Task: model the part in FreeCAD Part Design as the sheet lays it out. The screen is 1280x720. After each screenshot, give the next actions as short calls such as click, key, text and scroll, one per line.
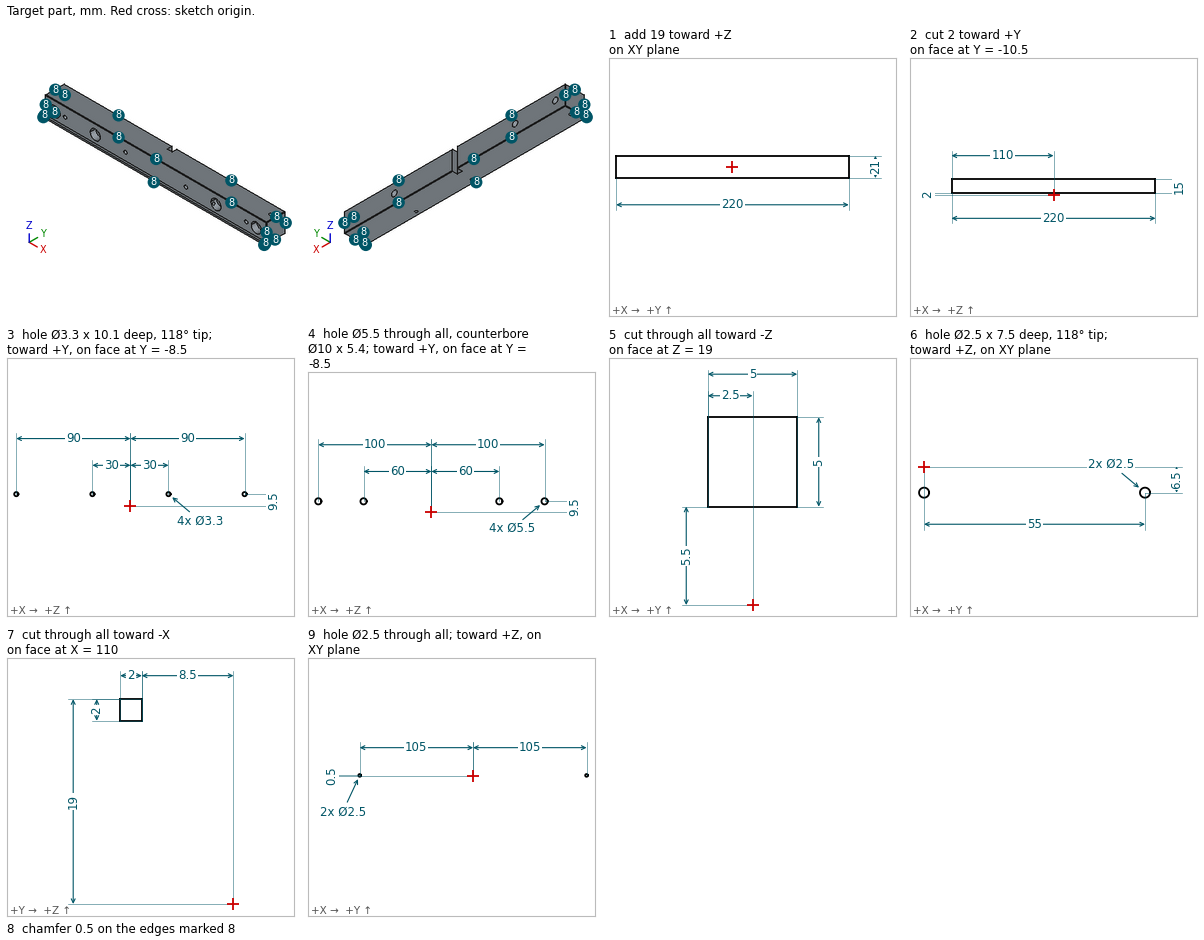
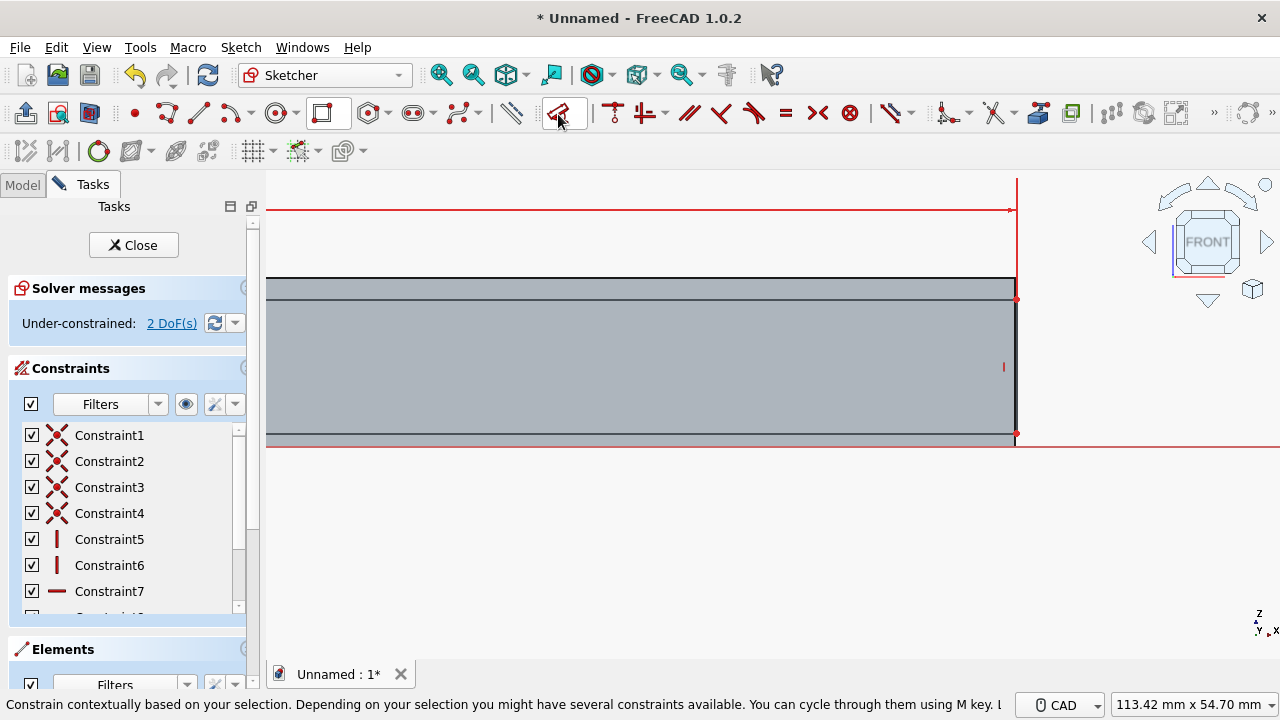
scroll(995, 433, down, 6)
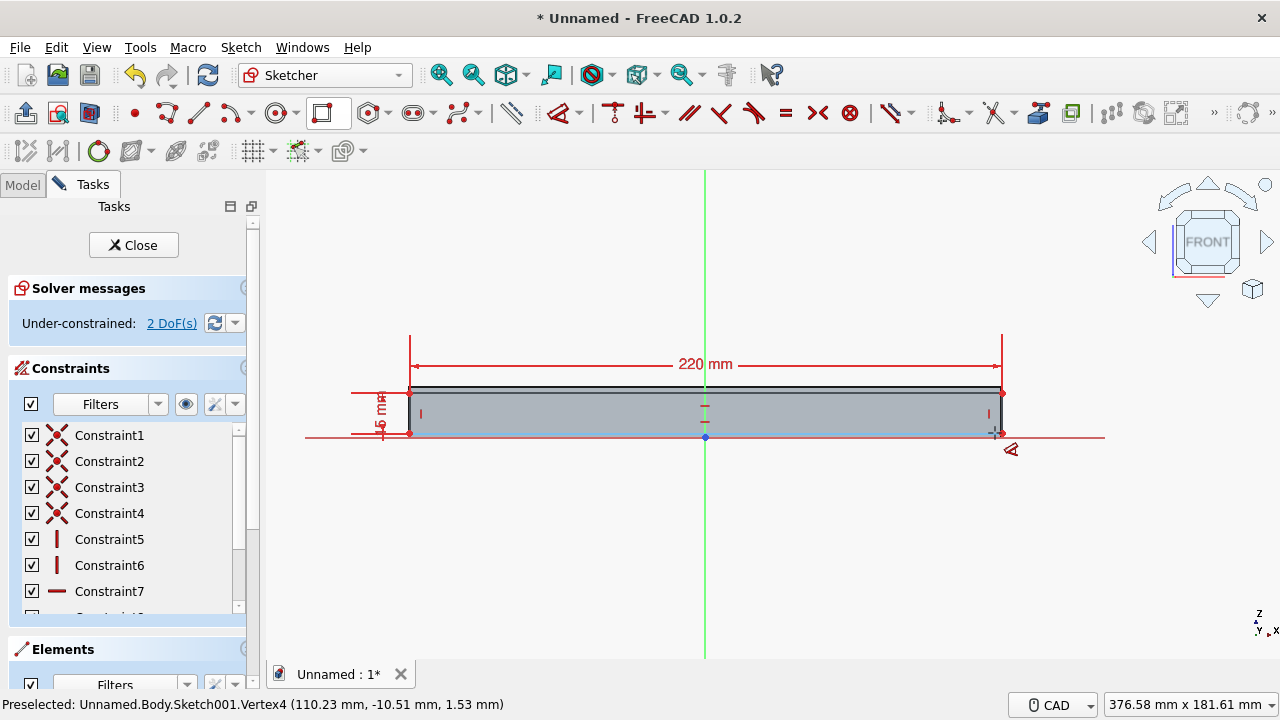
scroll(410, 434, up, 10)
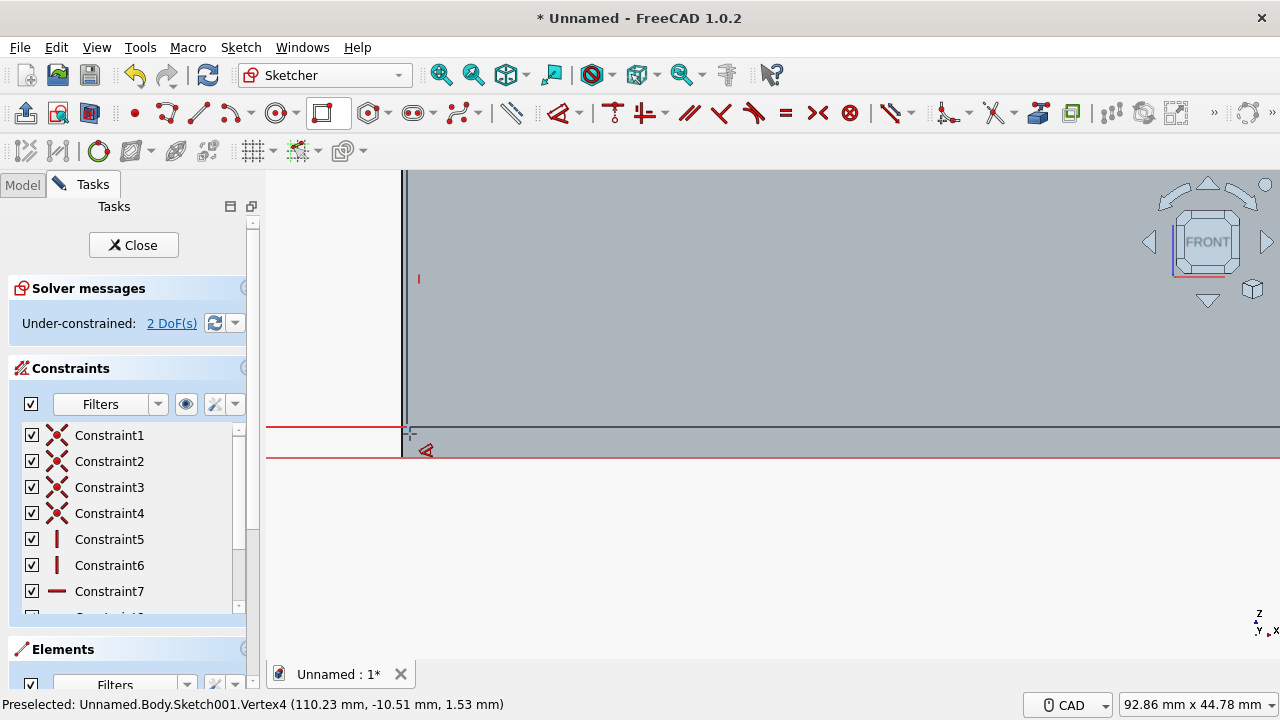
click(407, 427)
click(373, 443)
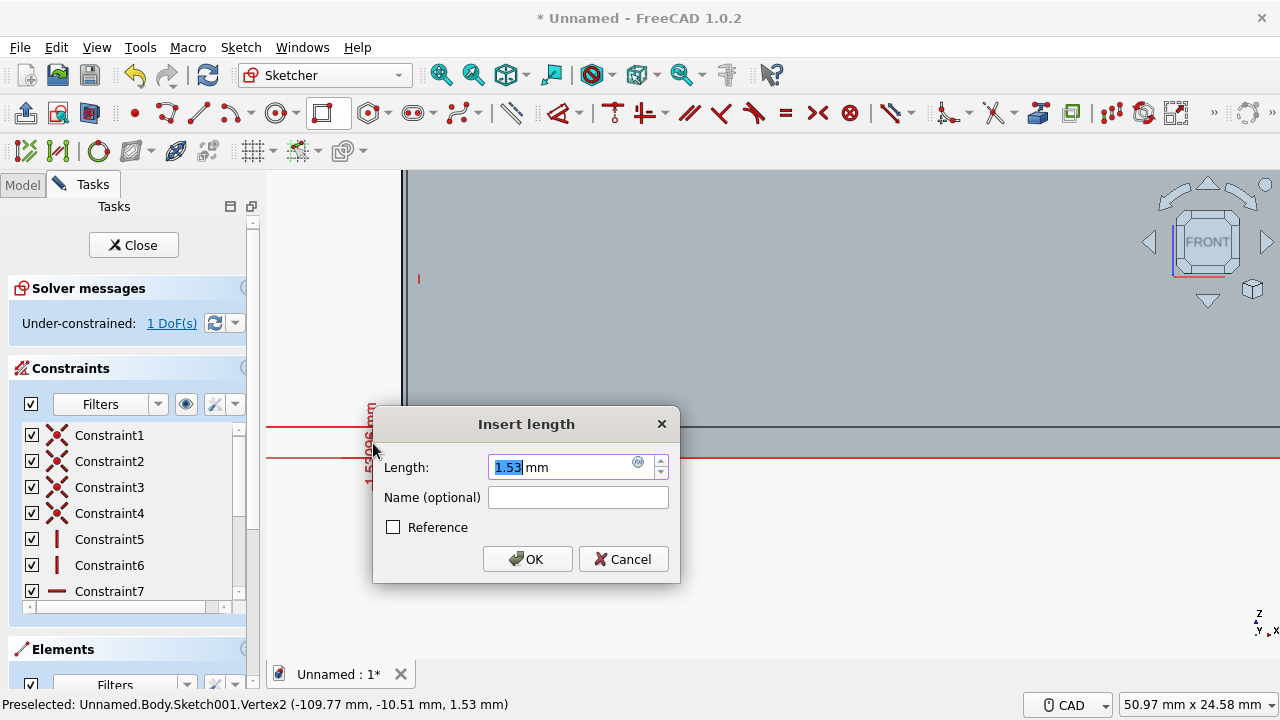
text(2)
key(Return)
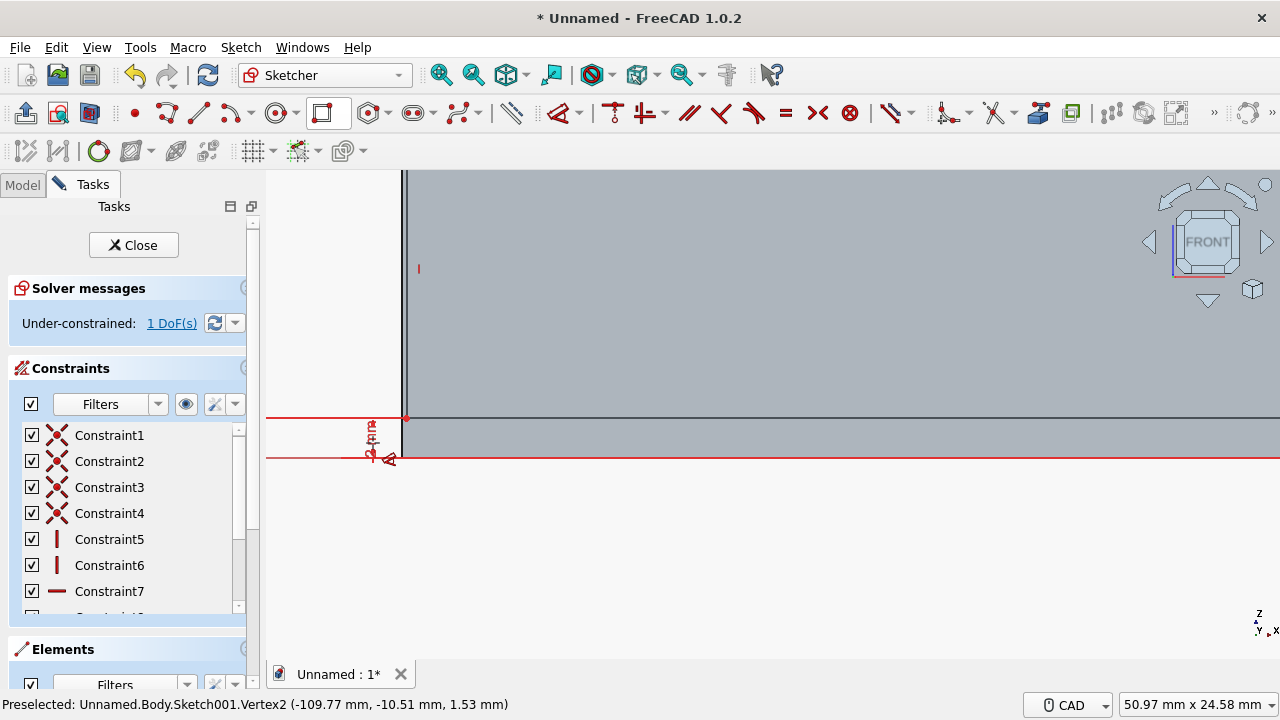
scroll(409, 434, down, 10)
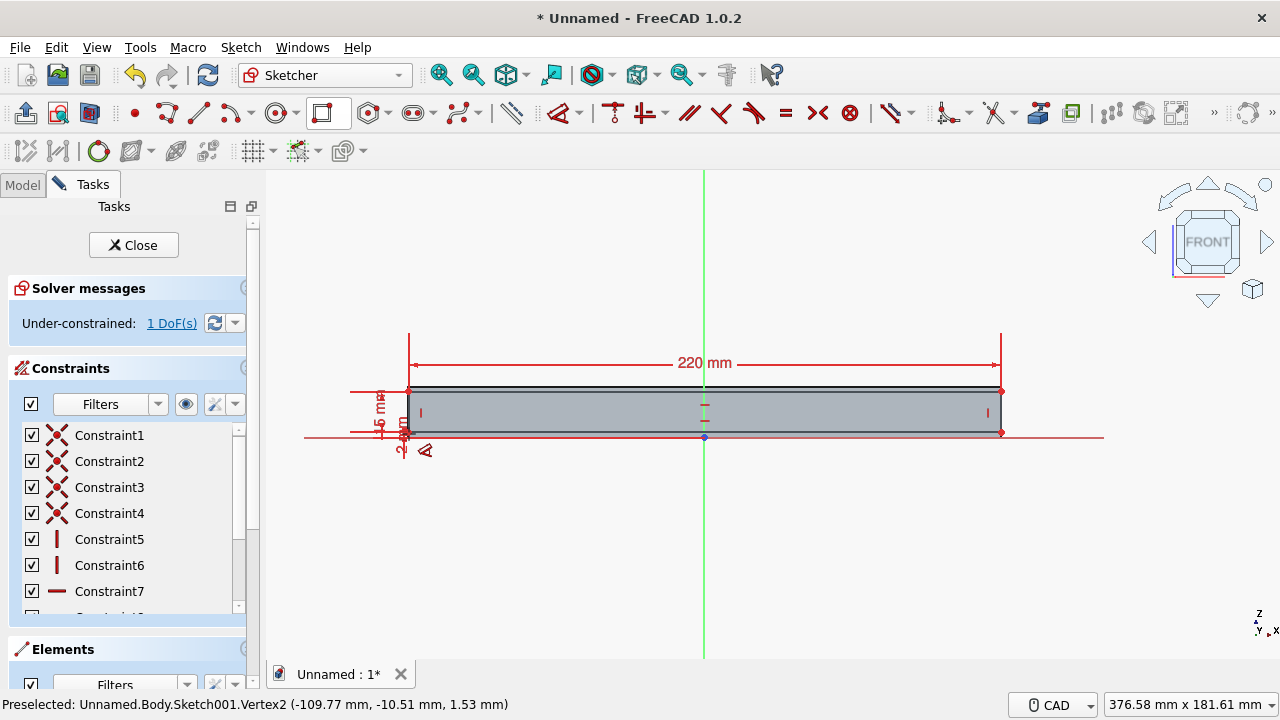
click(409, 392)
click(557, 472)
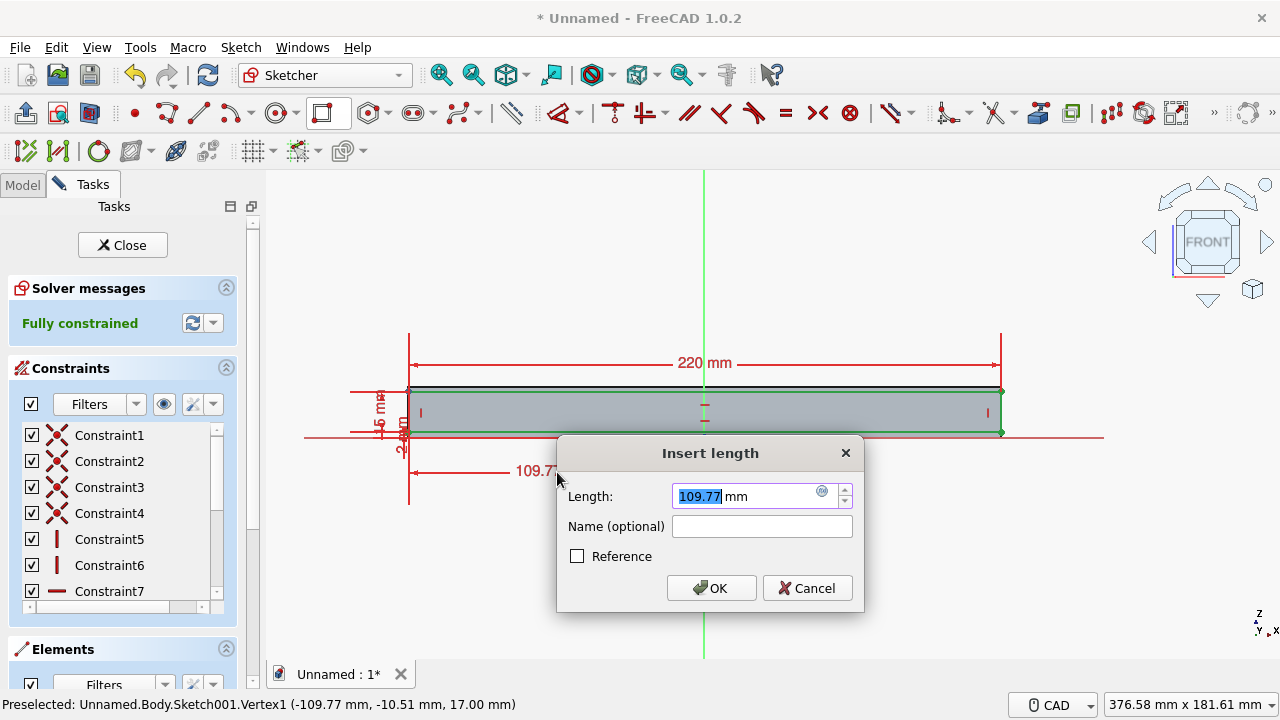
text(110)
key(Return)
key(Escape)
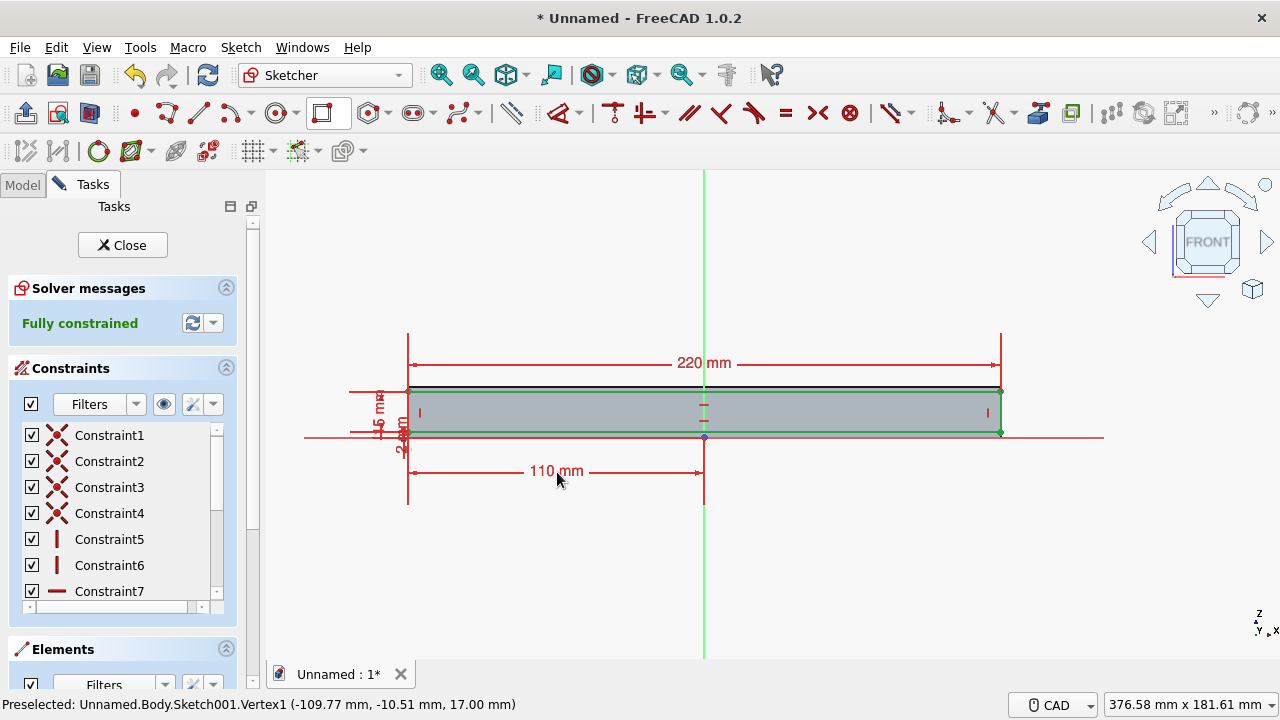
click(123, 245)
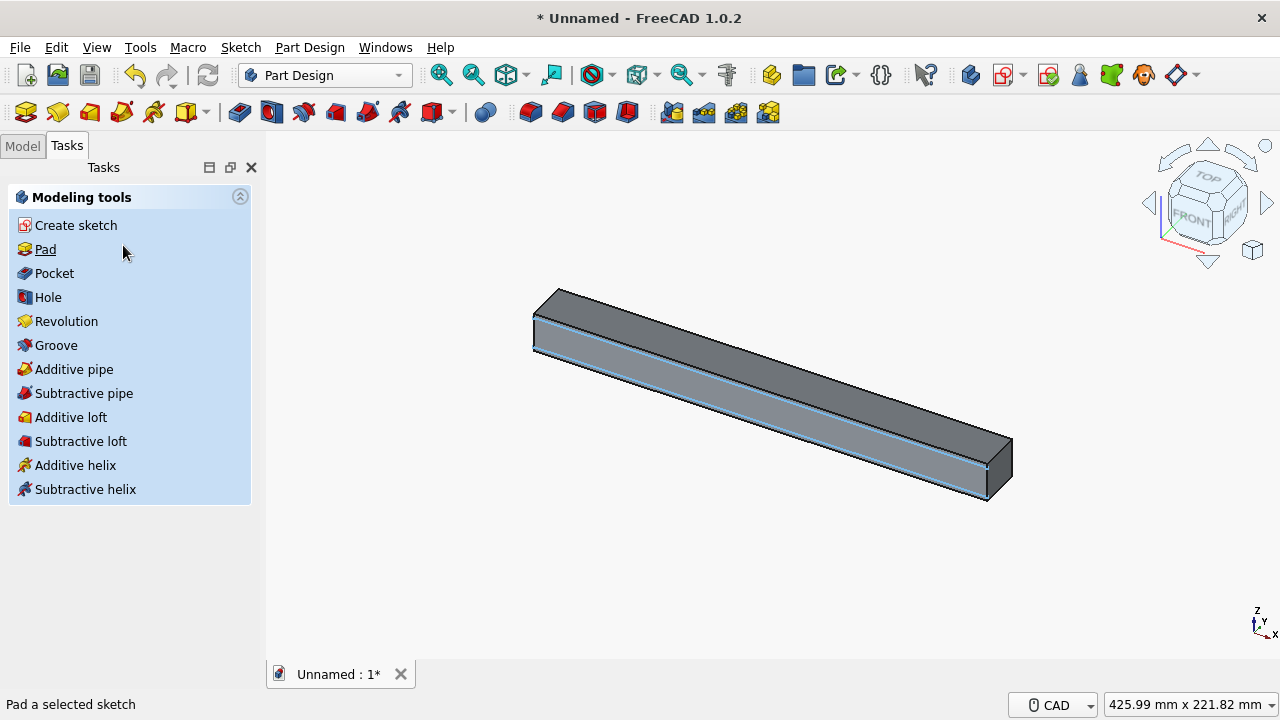
click(240, 112)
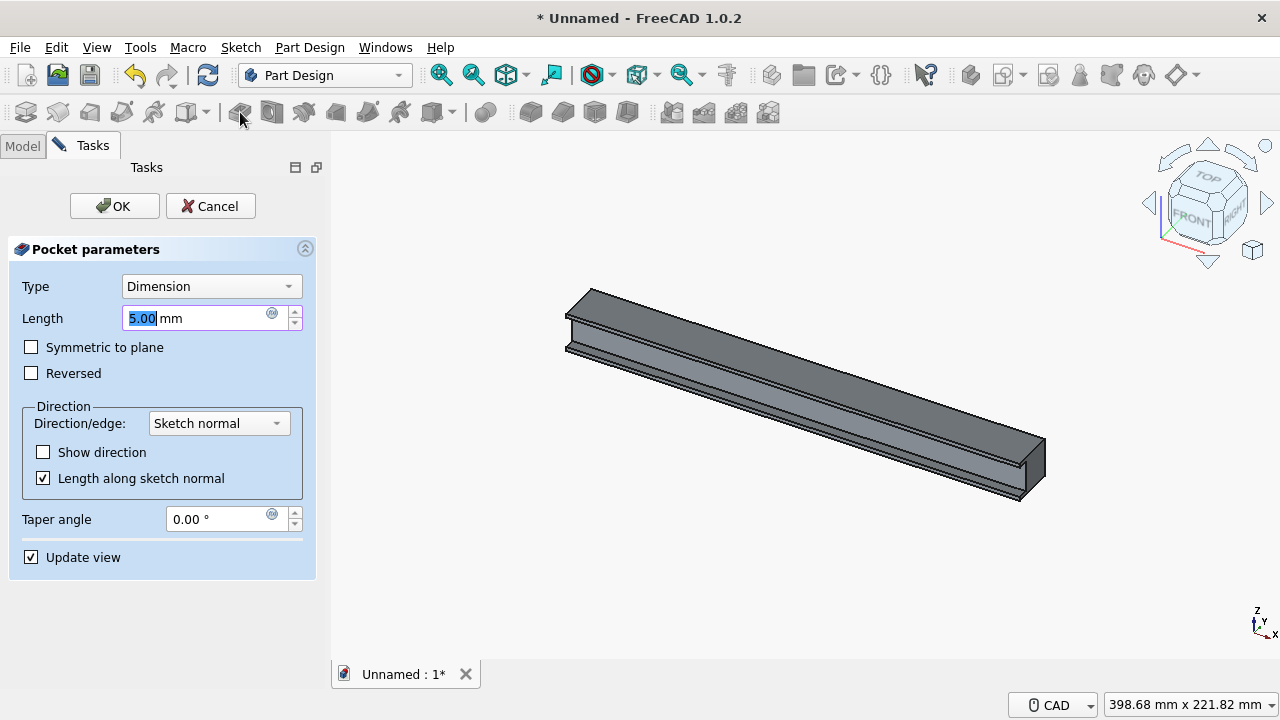
text(2)
key(Tab)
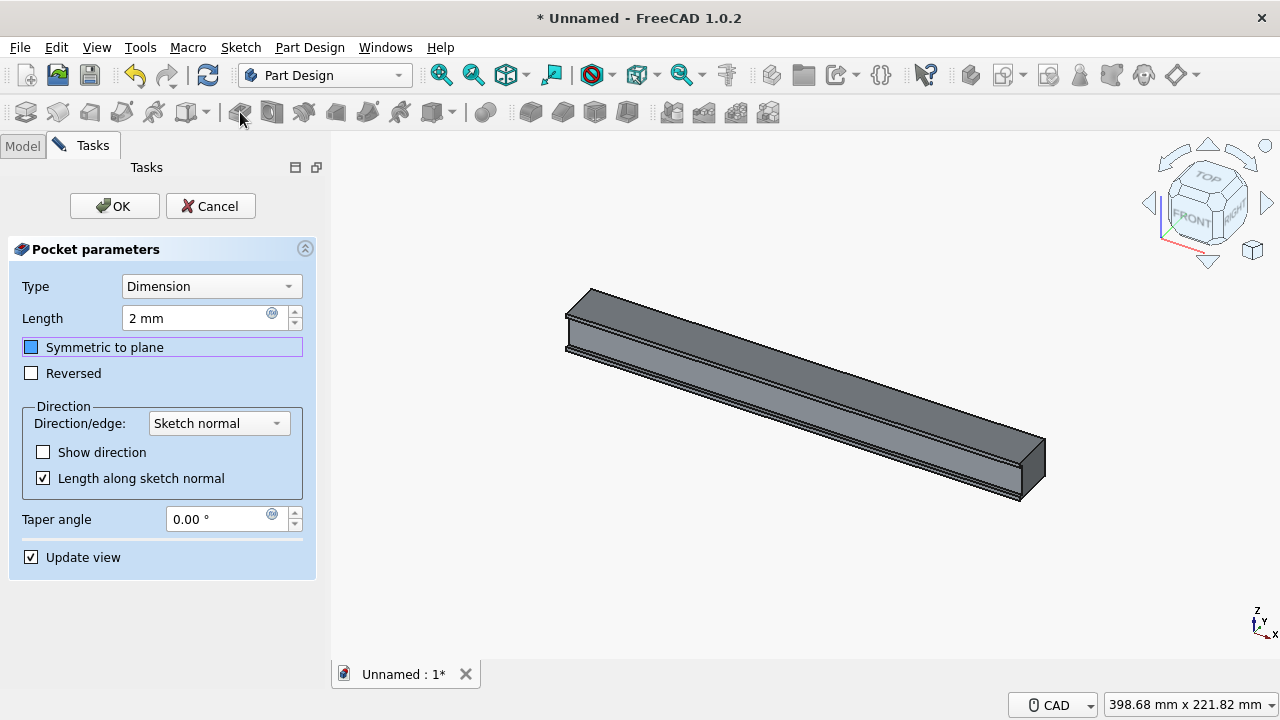
click(115, 206)